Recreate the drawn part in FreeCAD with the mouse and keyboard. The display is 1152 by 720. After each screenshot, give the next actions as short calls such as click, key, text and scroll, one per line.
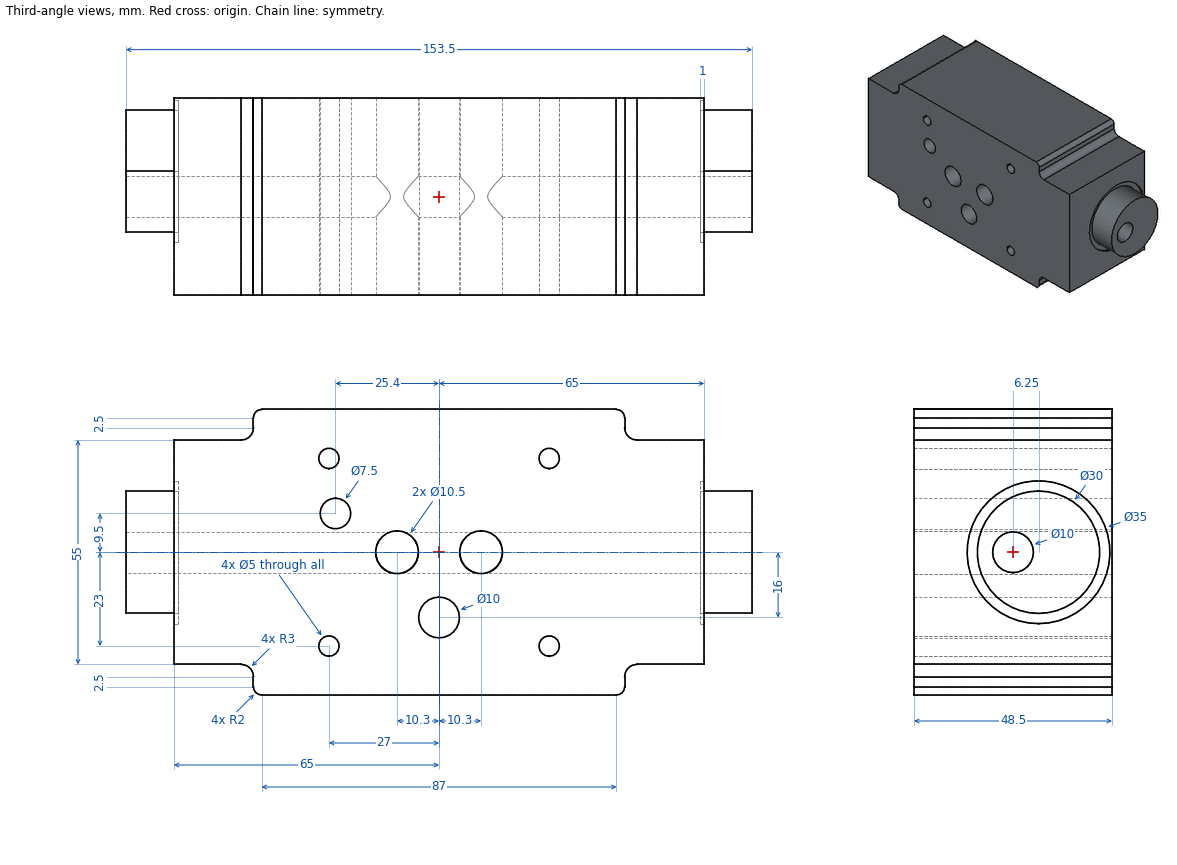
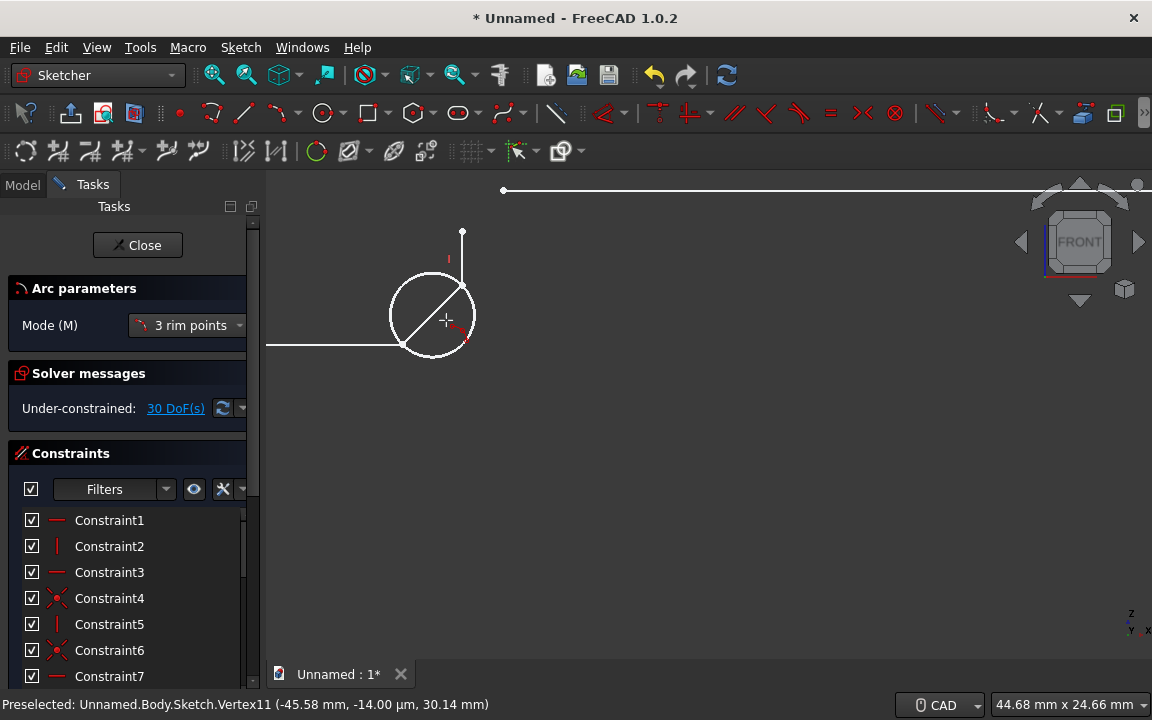
click(446, 320)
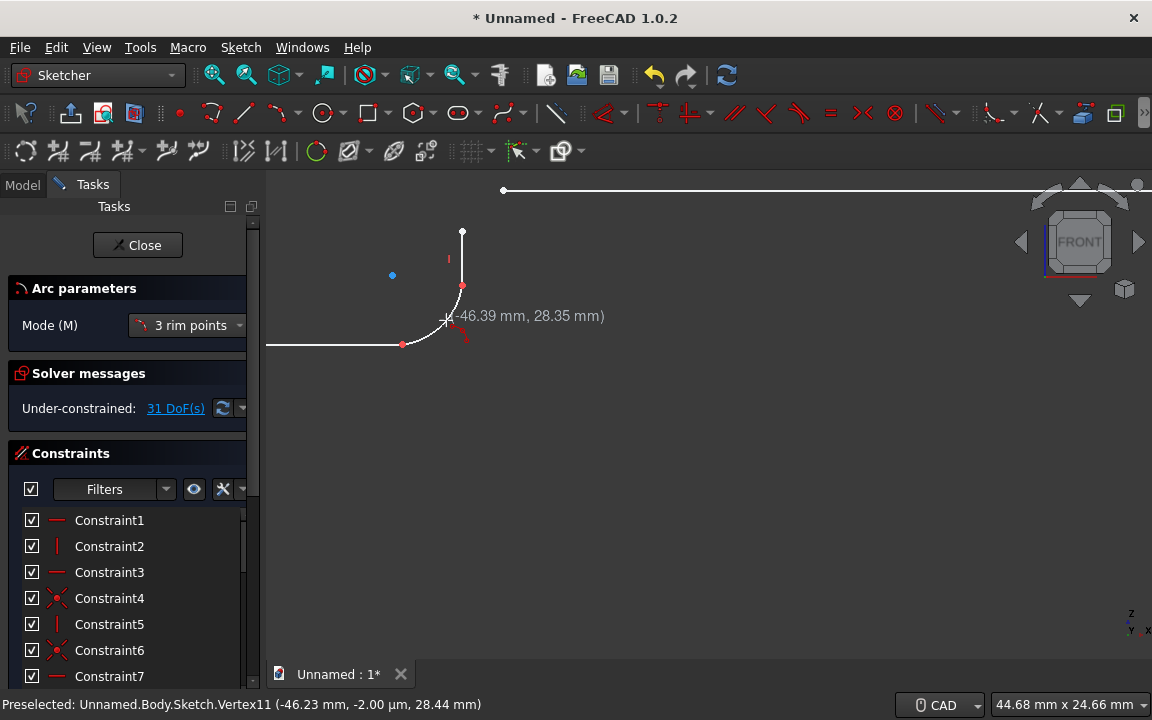
click(462, 231)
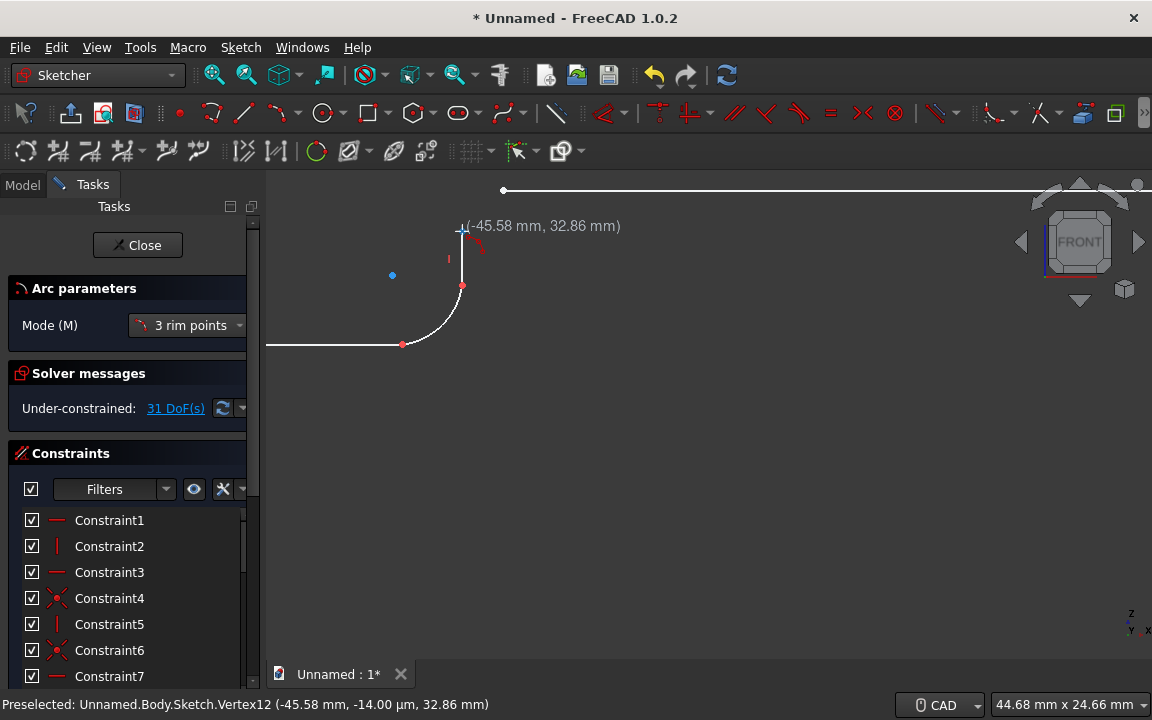
scroll(457, 296, down, 8)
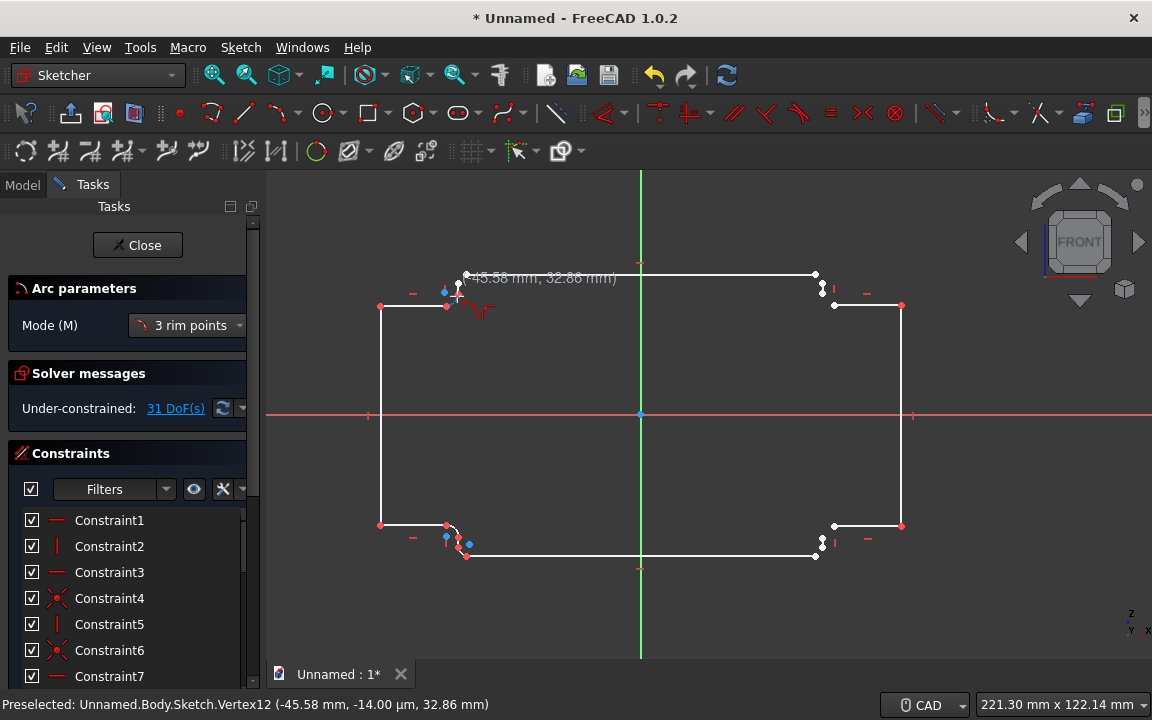
scroll(467, 275, up, 2)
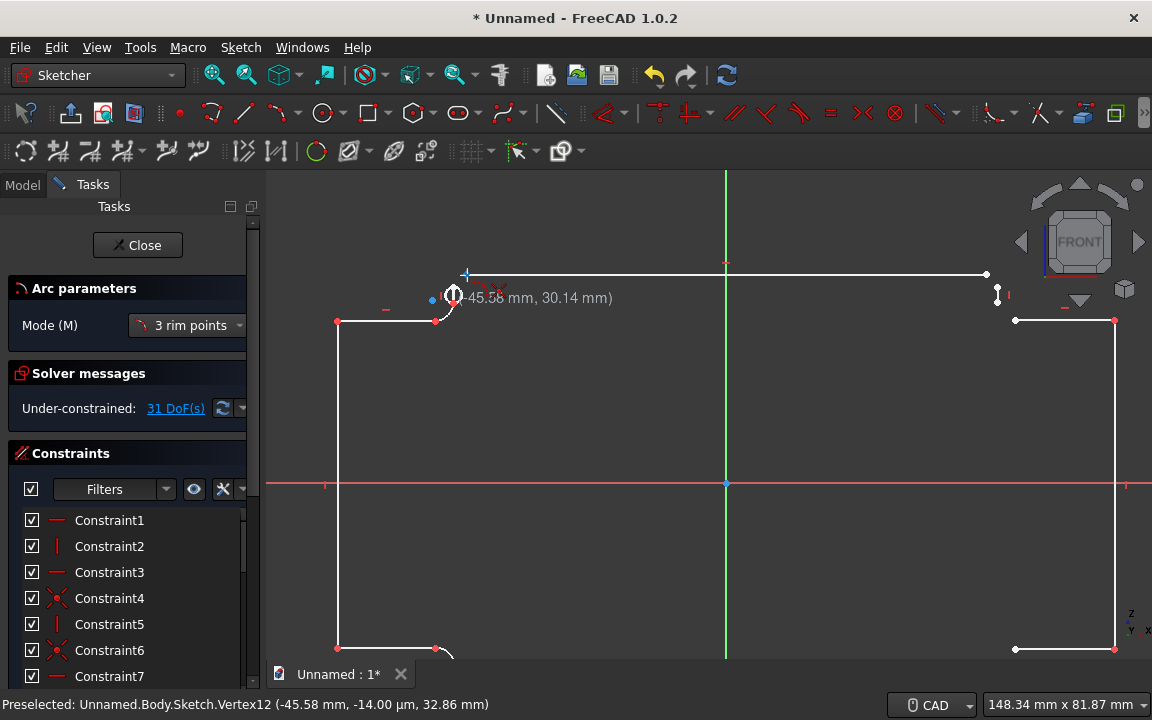
click(466, 275)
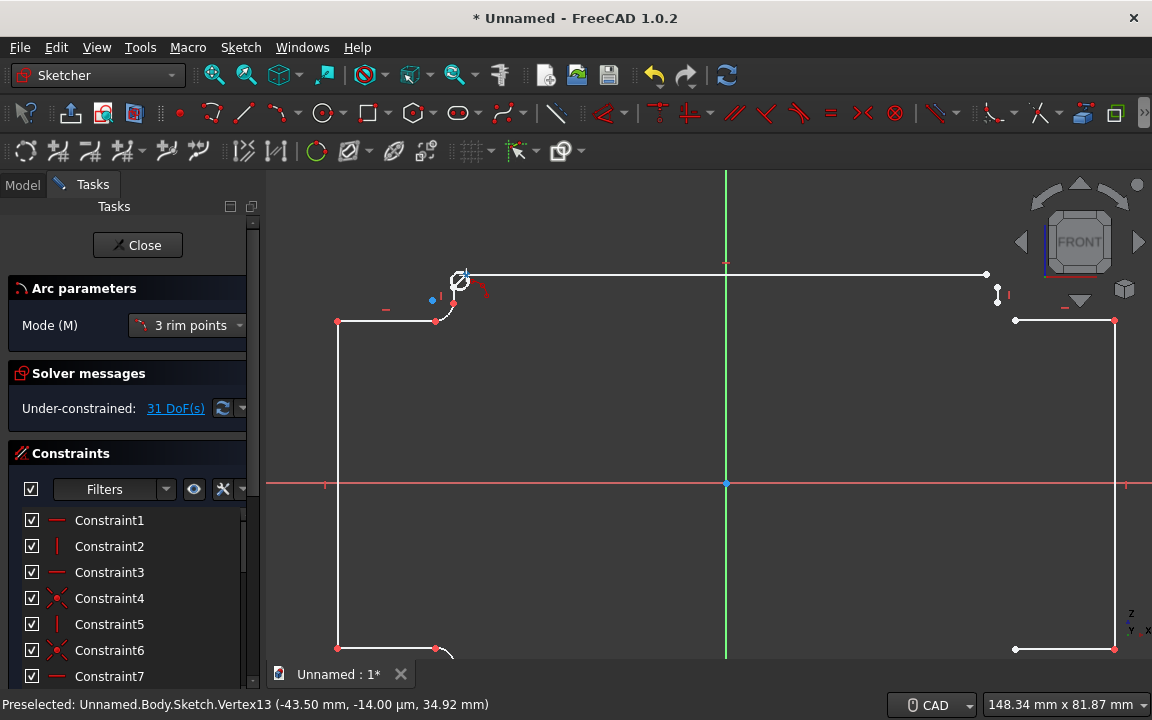
scroll(458, 278, up, 8)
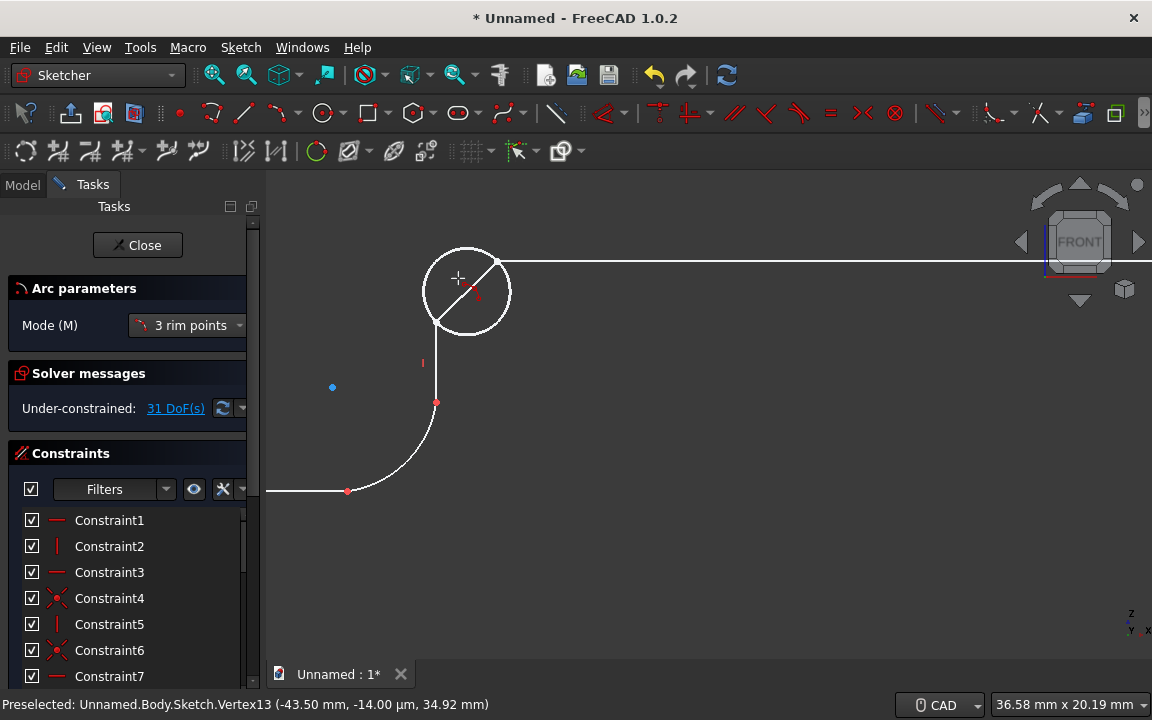
click(456, 276)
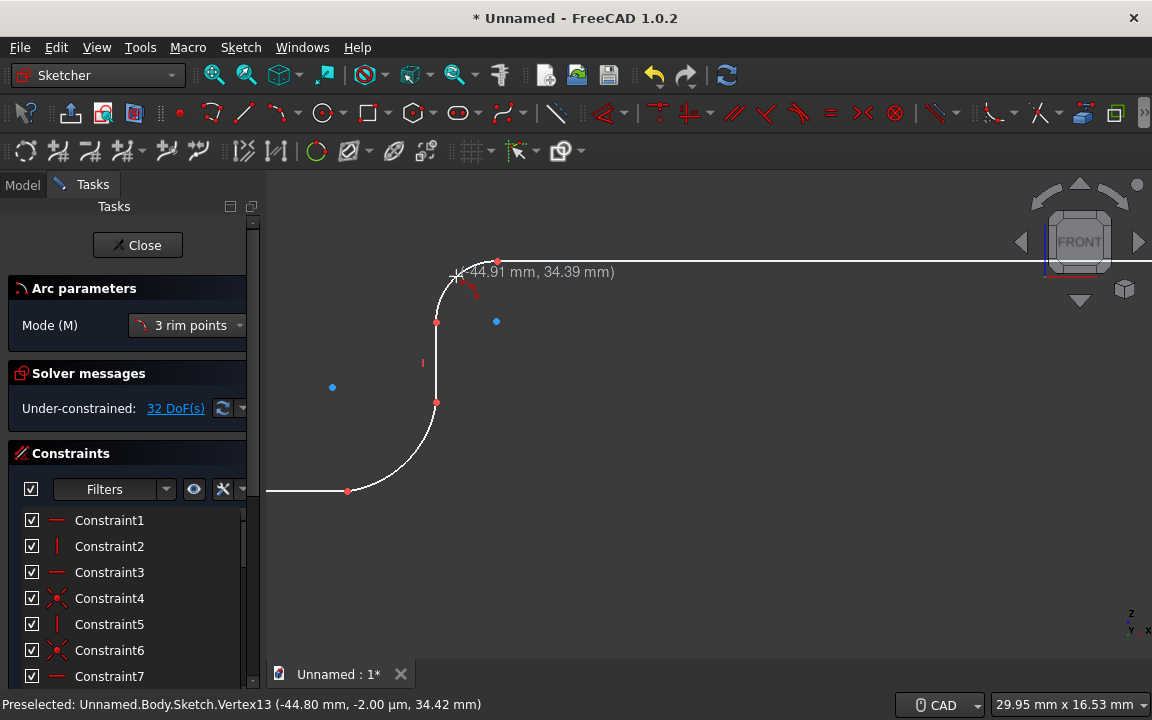
scroll(461, 277, down, 10)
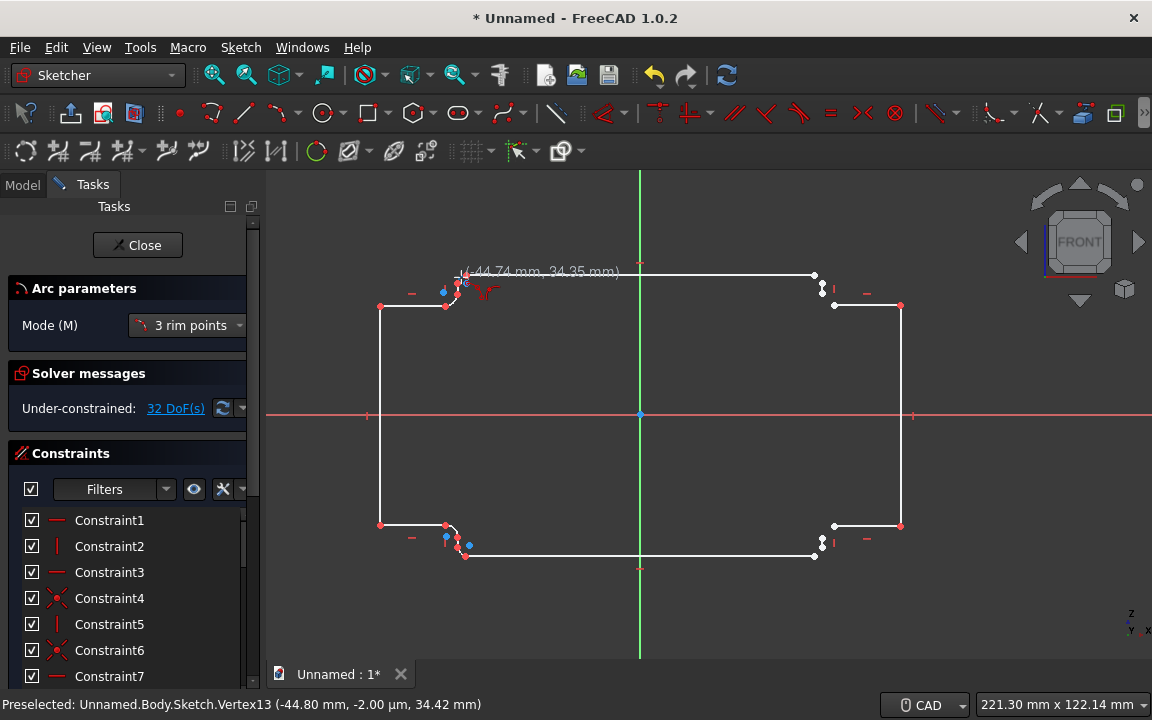
scroll(814, 275, up, 2)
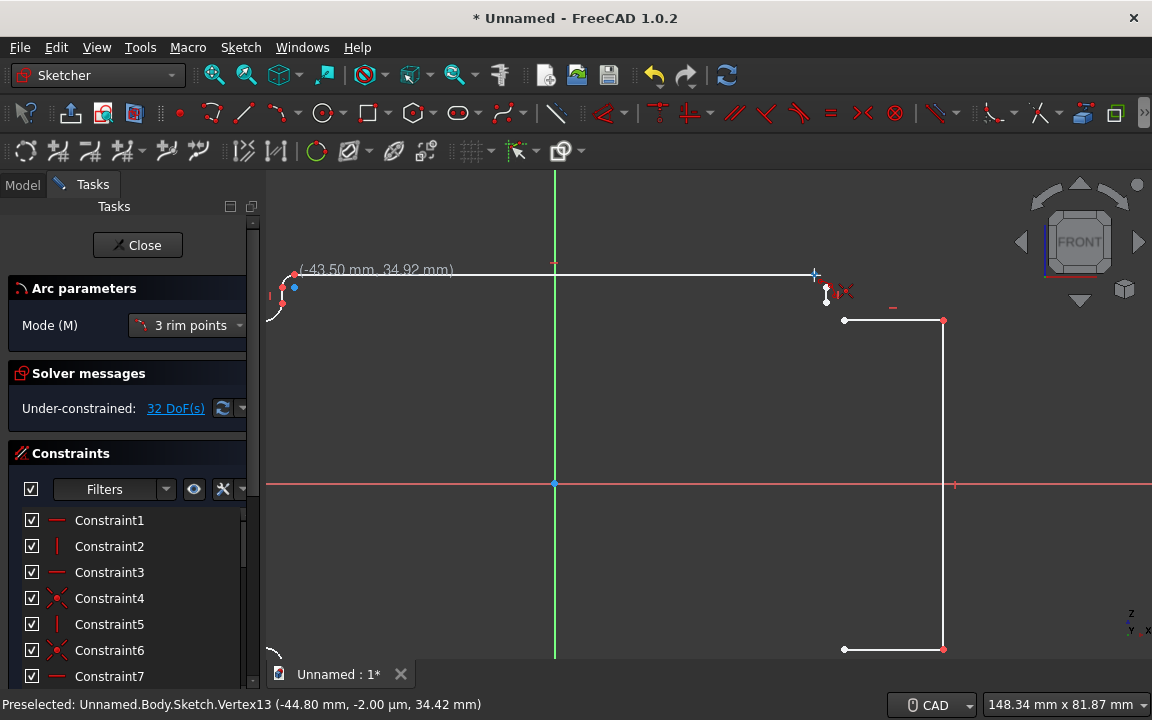
click(815, 275)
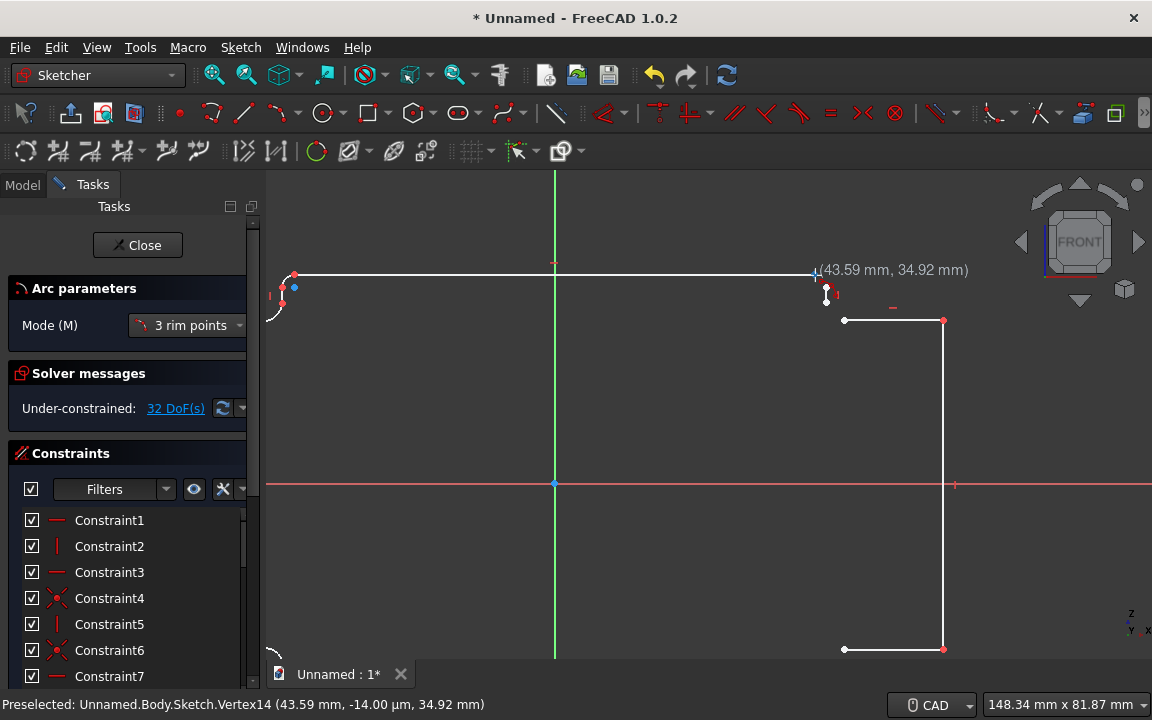
scroll(826, 286, up, 4)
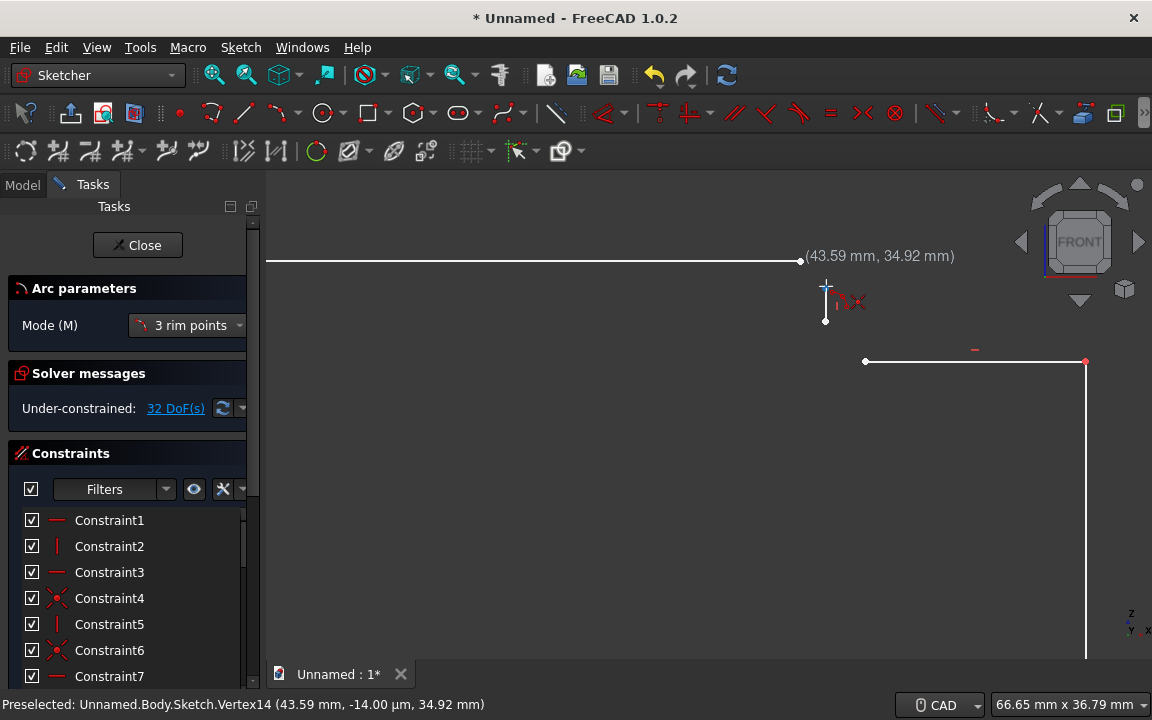
click(826, 288)